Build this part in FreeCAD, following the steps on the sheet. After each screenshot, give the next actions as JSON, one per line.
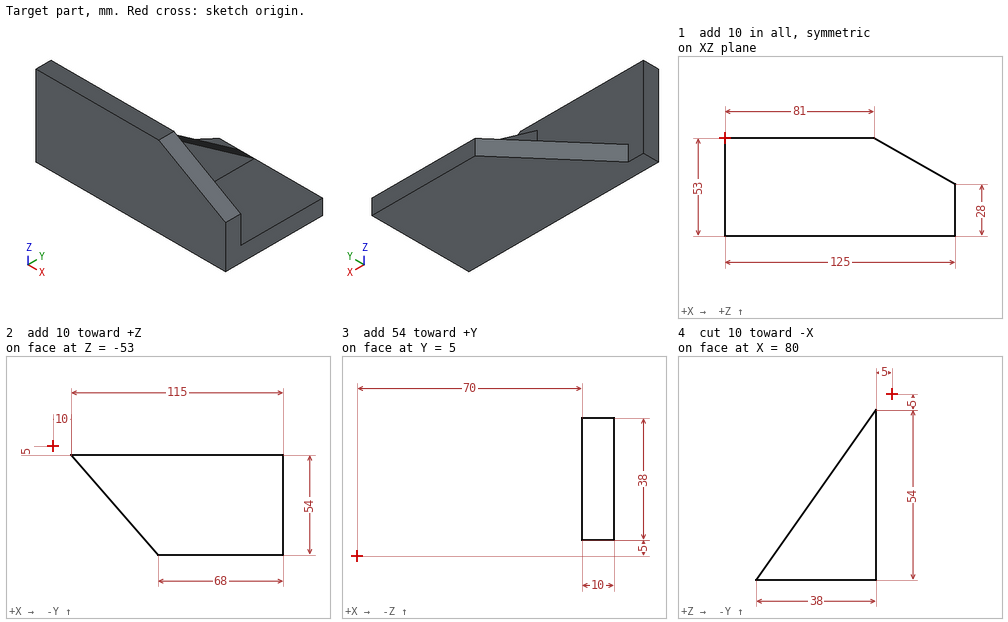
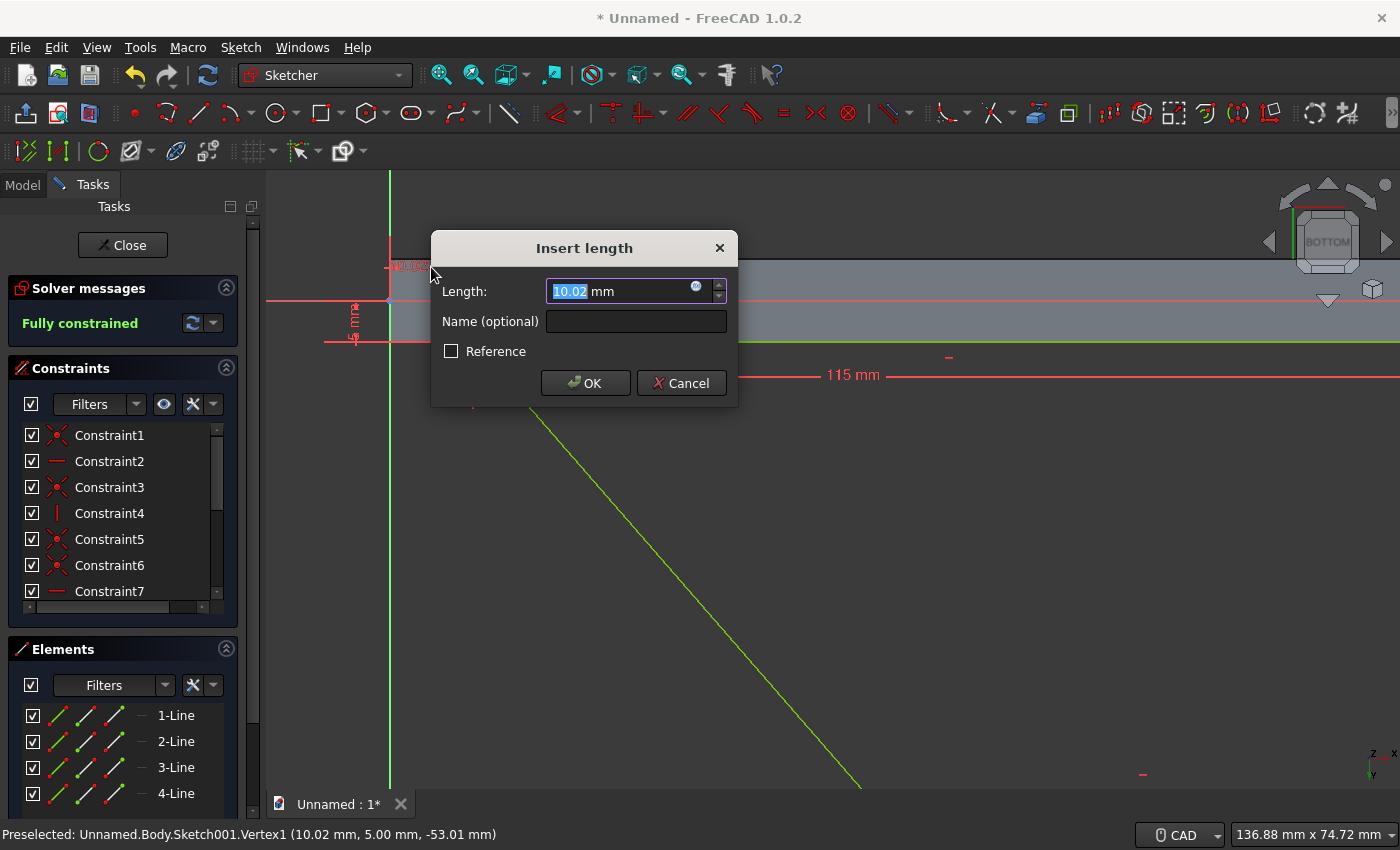
{"action": "type", "text": "10"}
{"action": "key", "text": "Return"}
{"action": "key", "text": "Escape"}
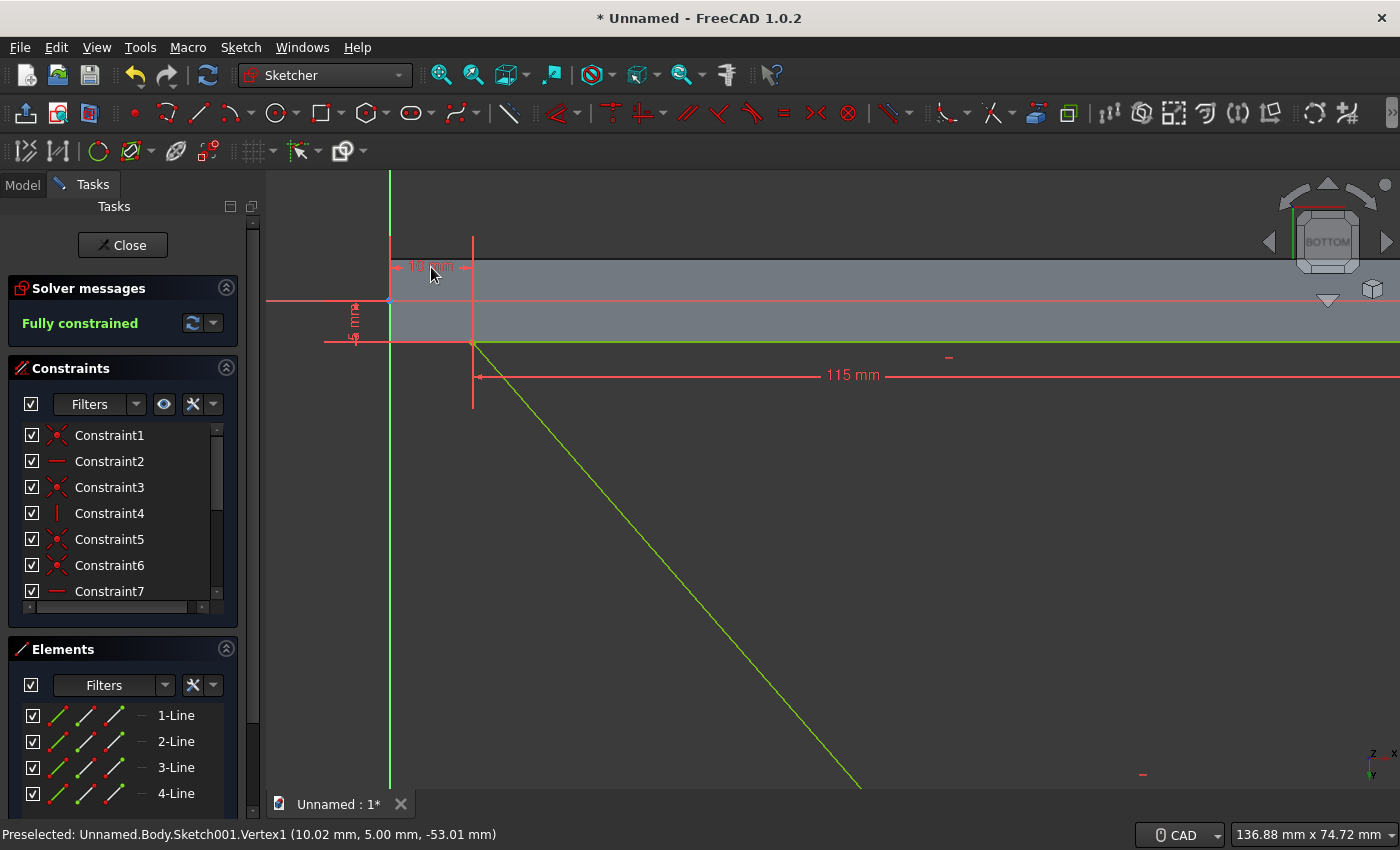
{"action": "left_click", "coordinate": [123, 245]}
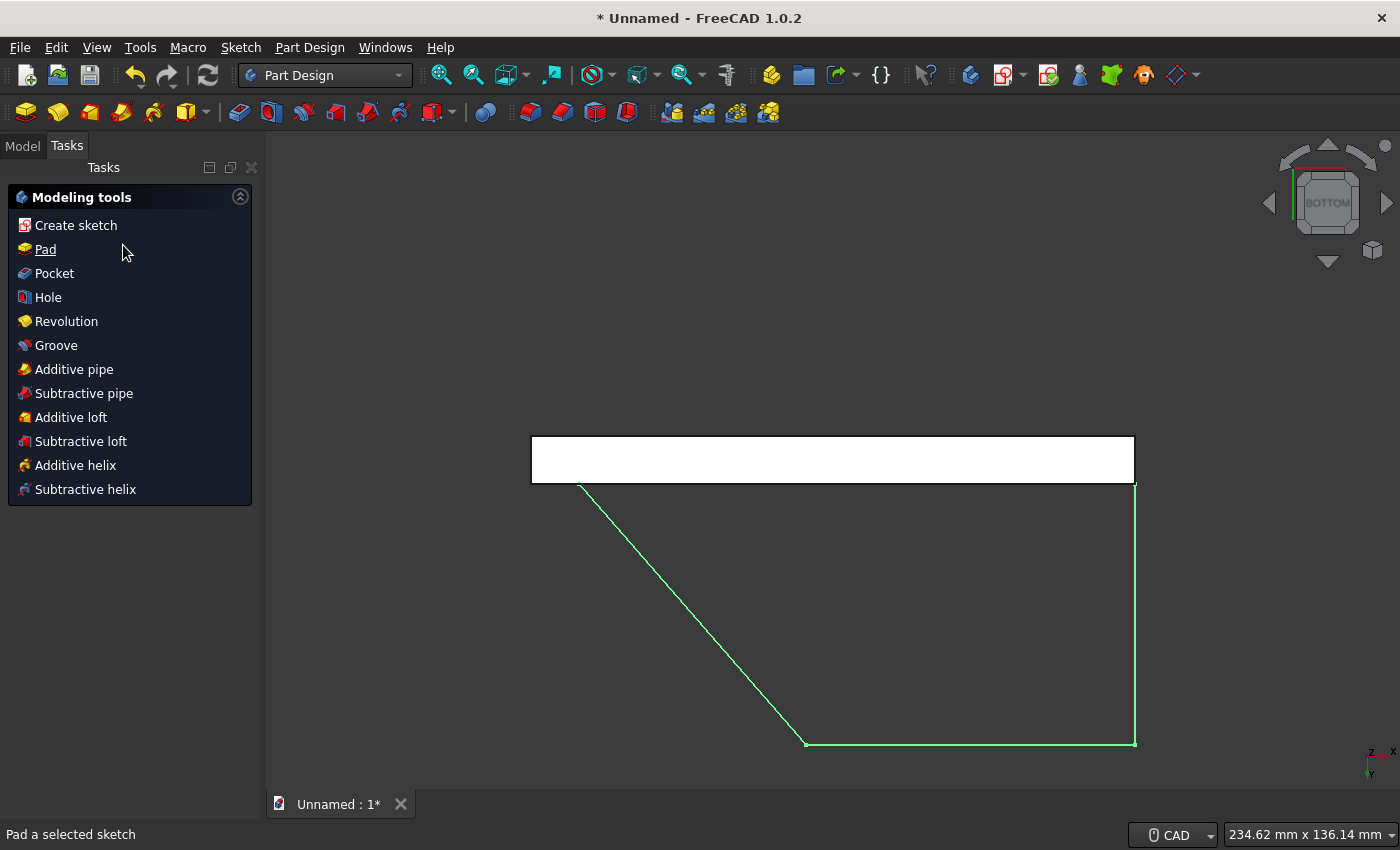
{"action": "left_click", "coordinate": [26, 112]}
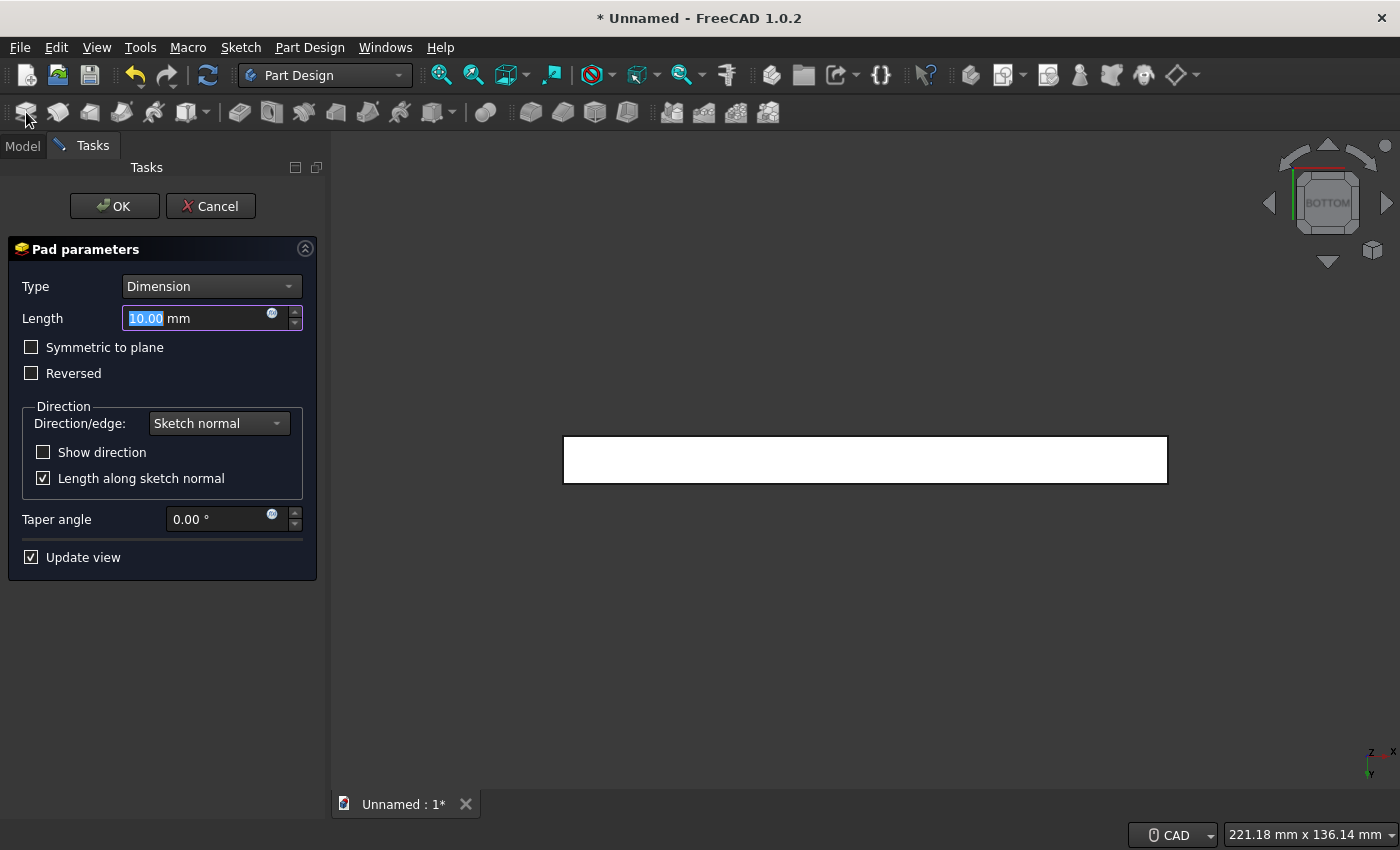
{"action": "type", "text": "10"}
{"action": "key", "text": "Tab"}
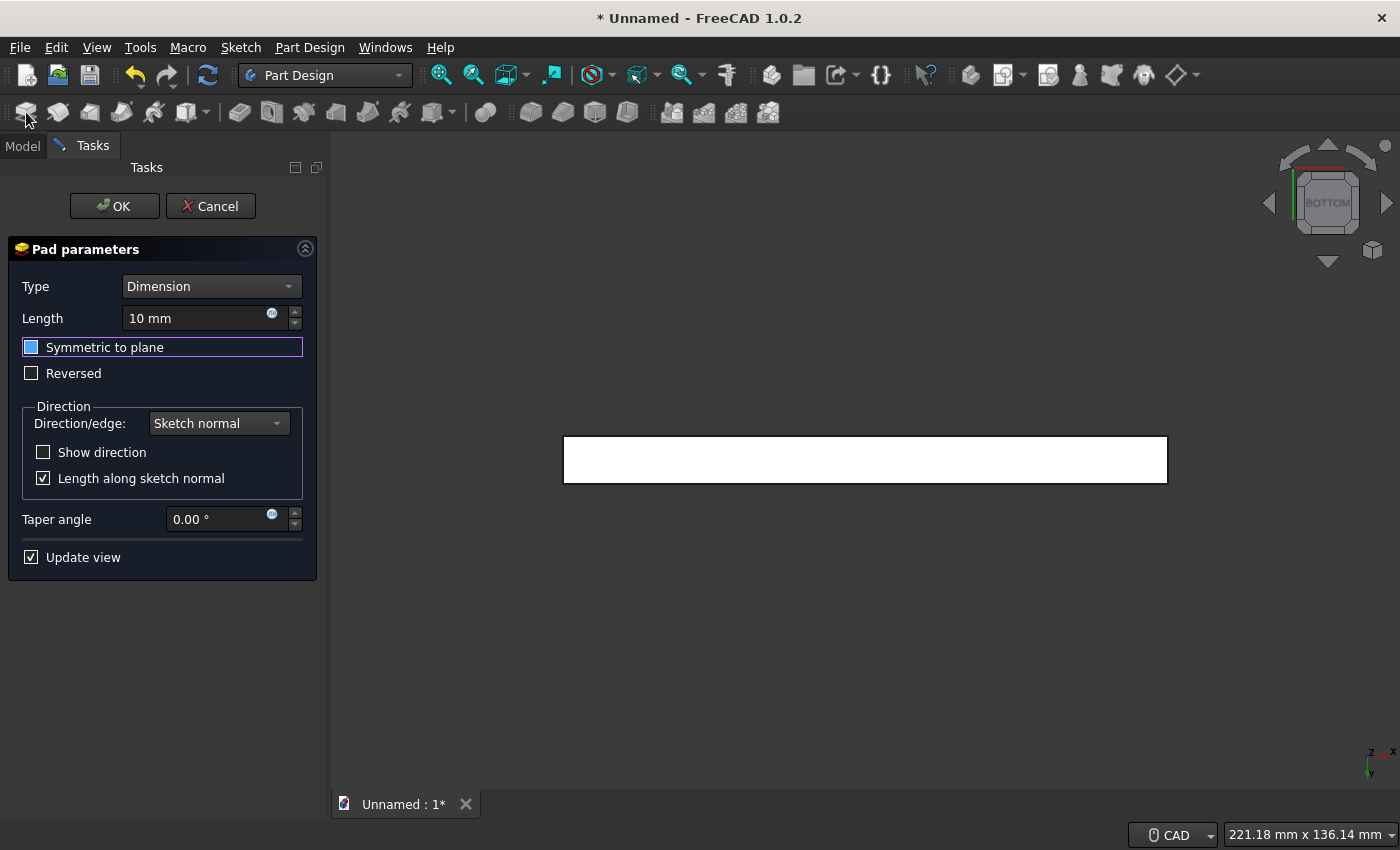
{"action": "left_click", "coordinate": [30, 373]}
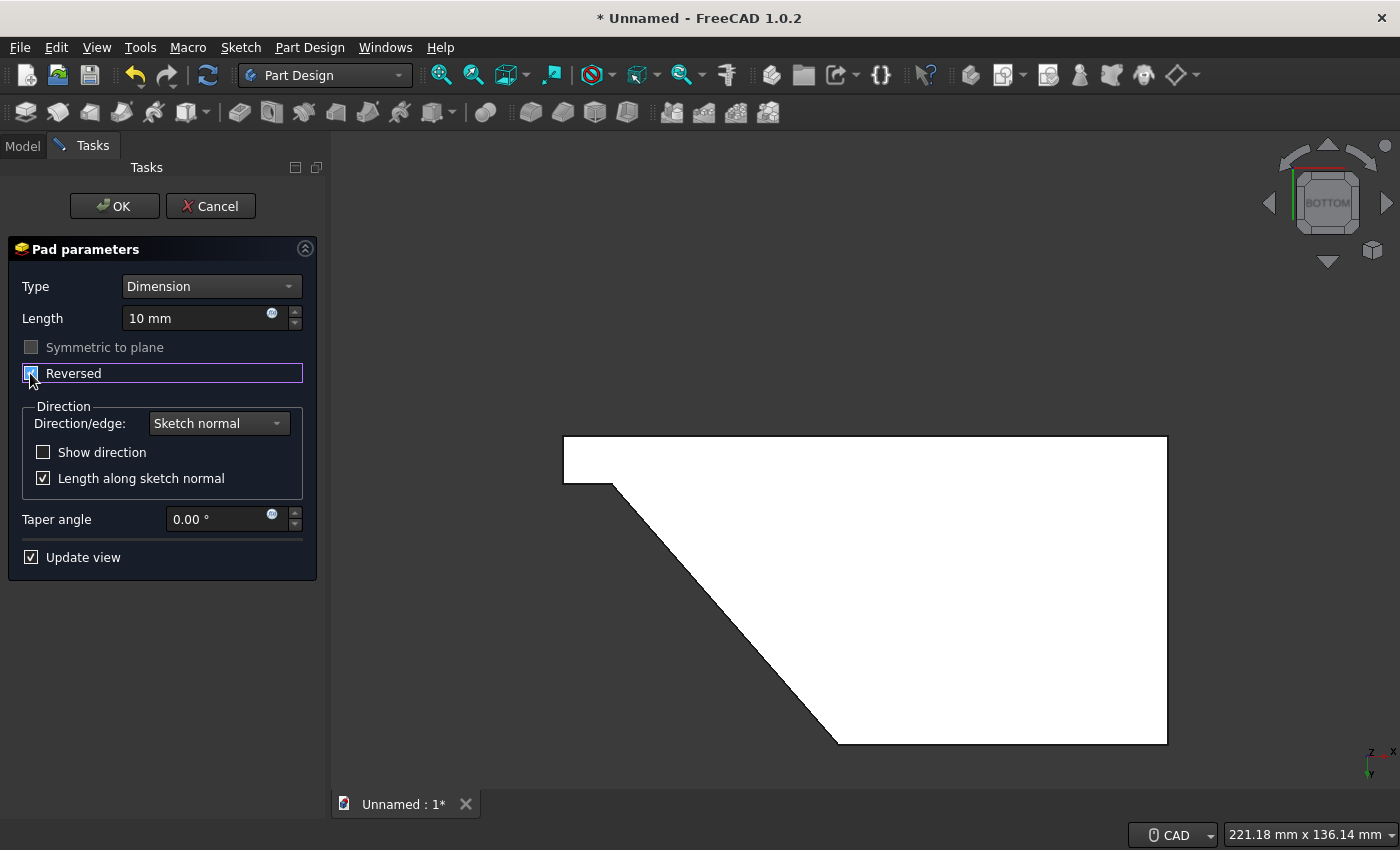
{"action": "left_click", "coordinate": [115, 206]}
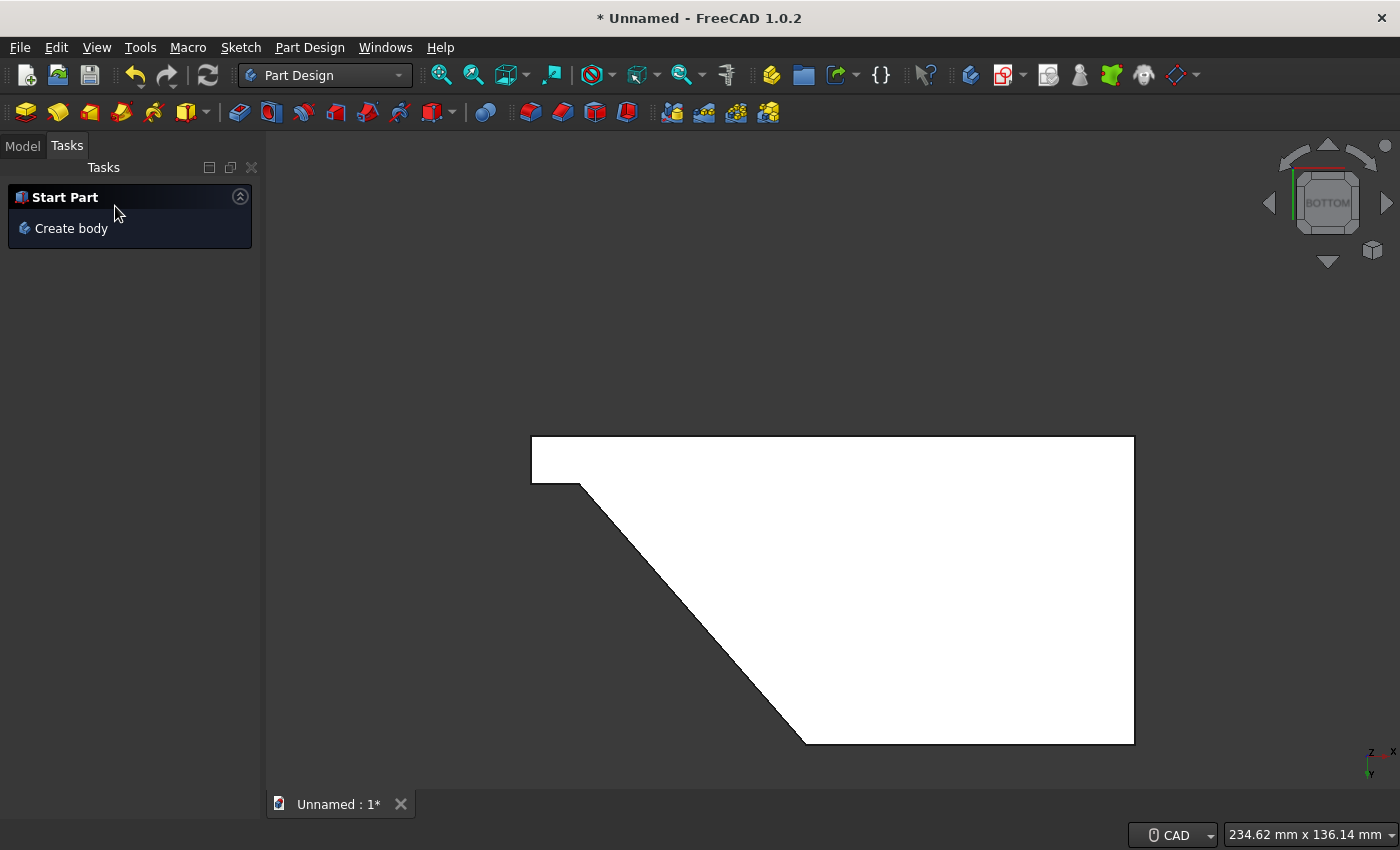
{"action": "key", "text": "4"}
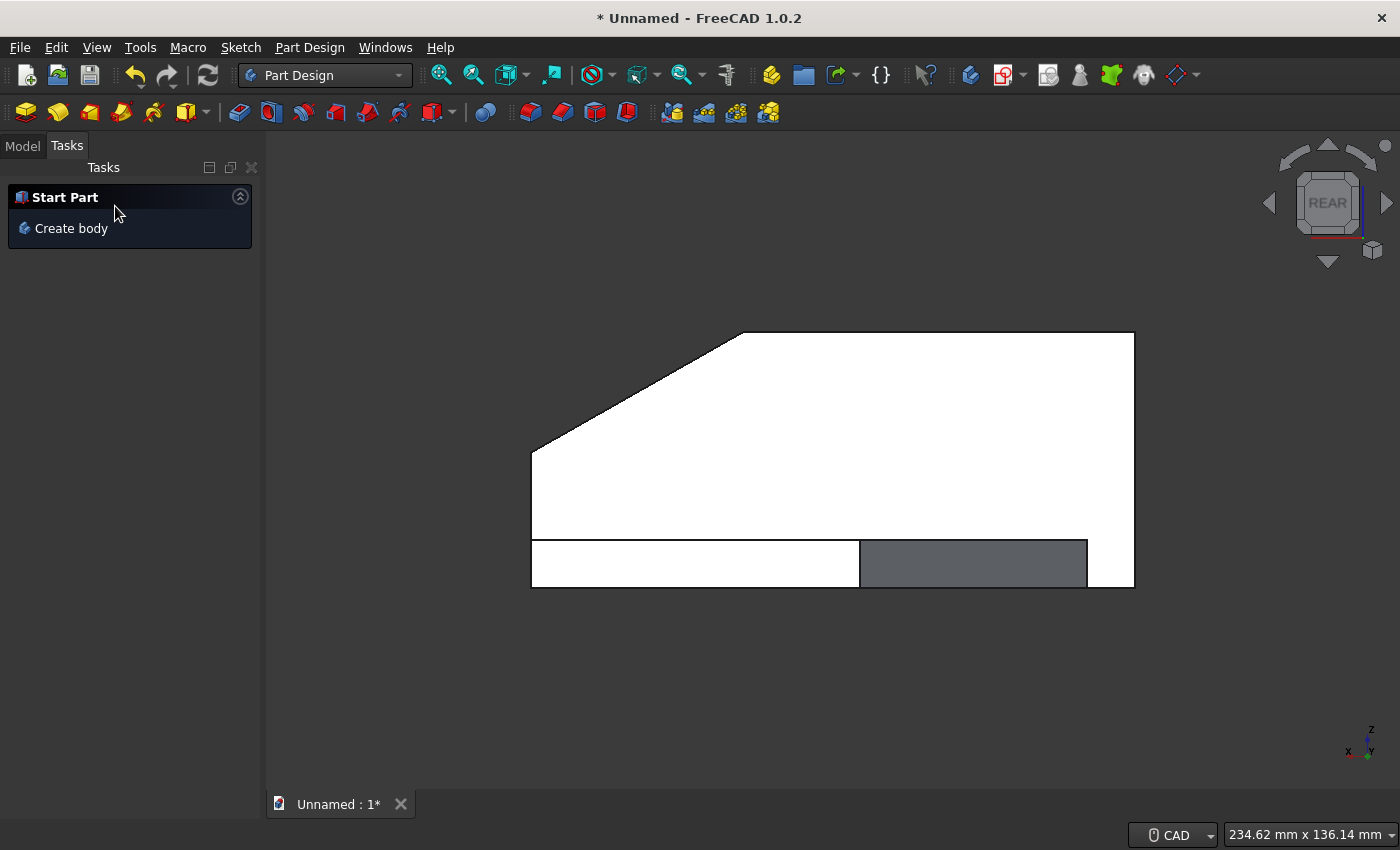
{"action": "left_click", "coordinate": [833, 422]}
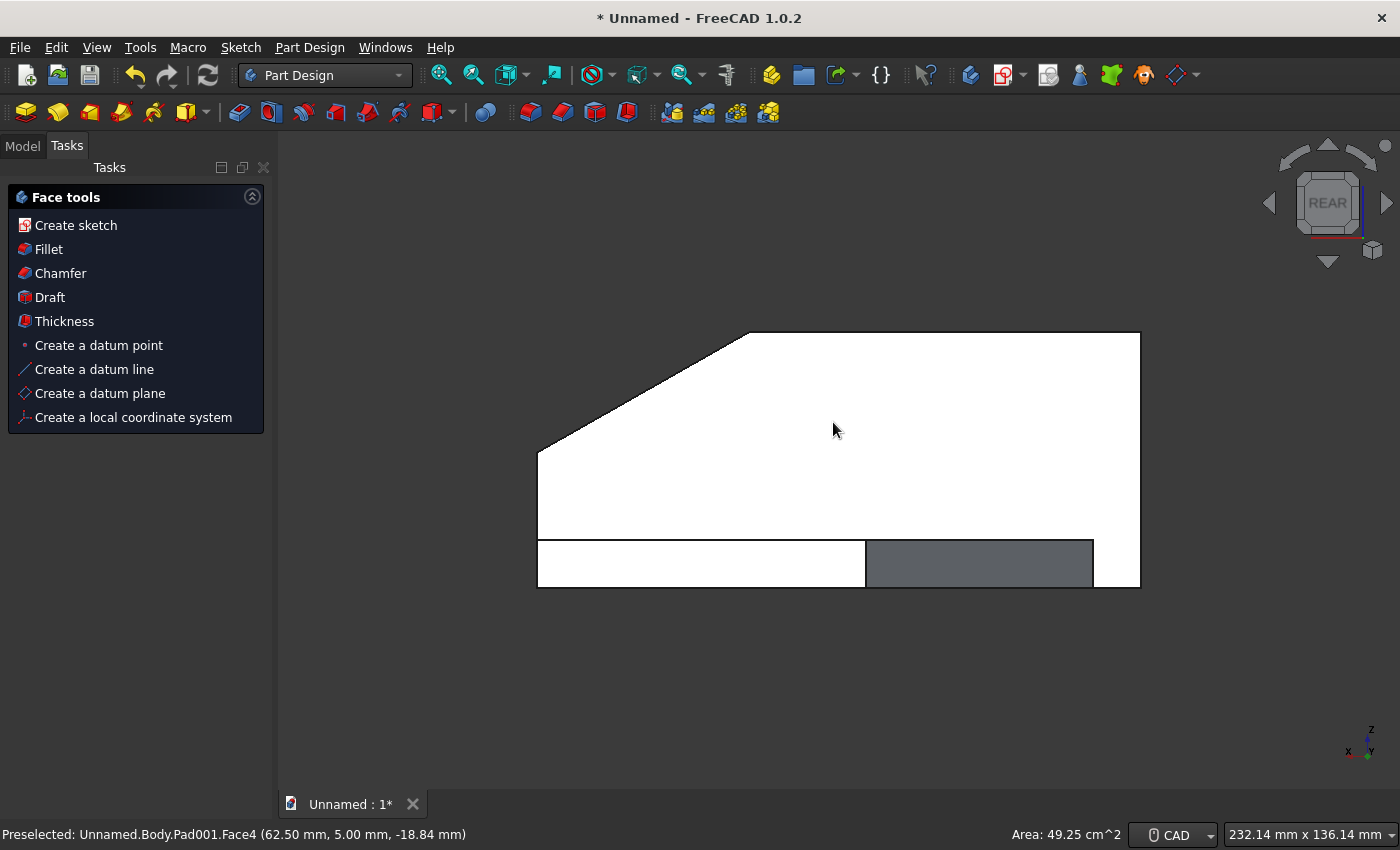
{"action": "left_click", "coordinate": [1004, 76]}